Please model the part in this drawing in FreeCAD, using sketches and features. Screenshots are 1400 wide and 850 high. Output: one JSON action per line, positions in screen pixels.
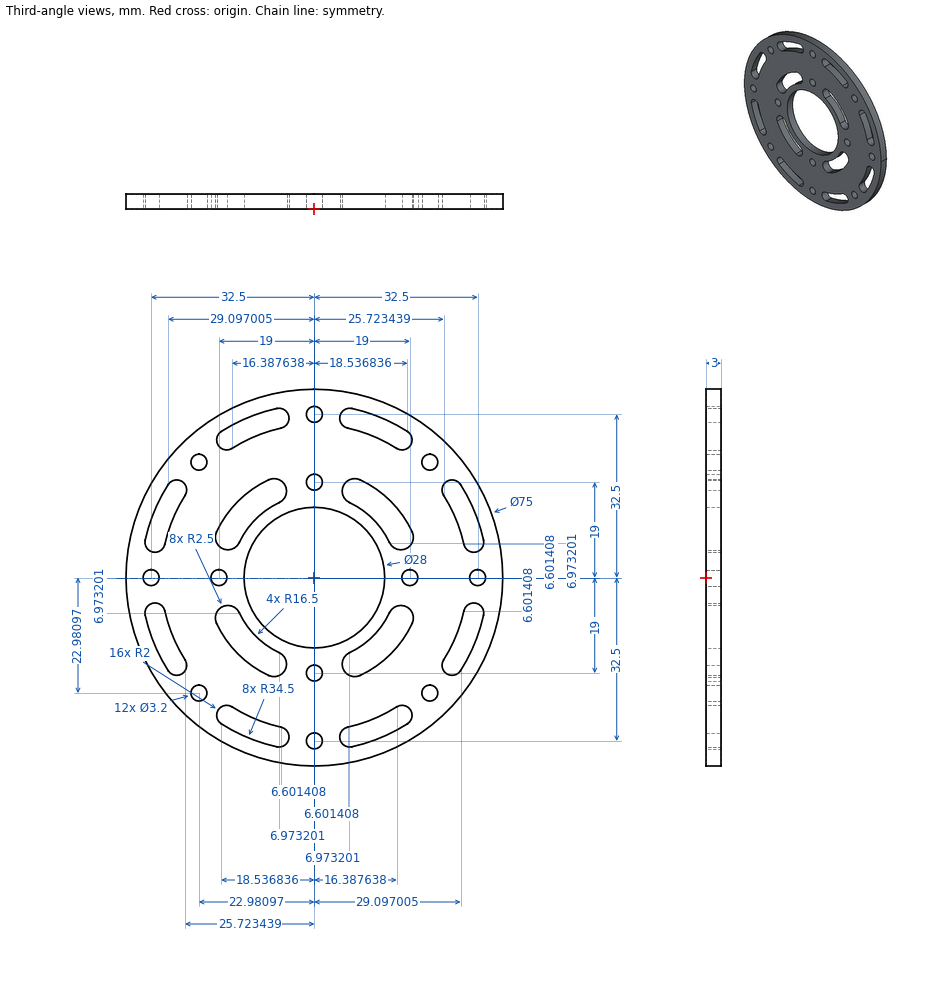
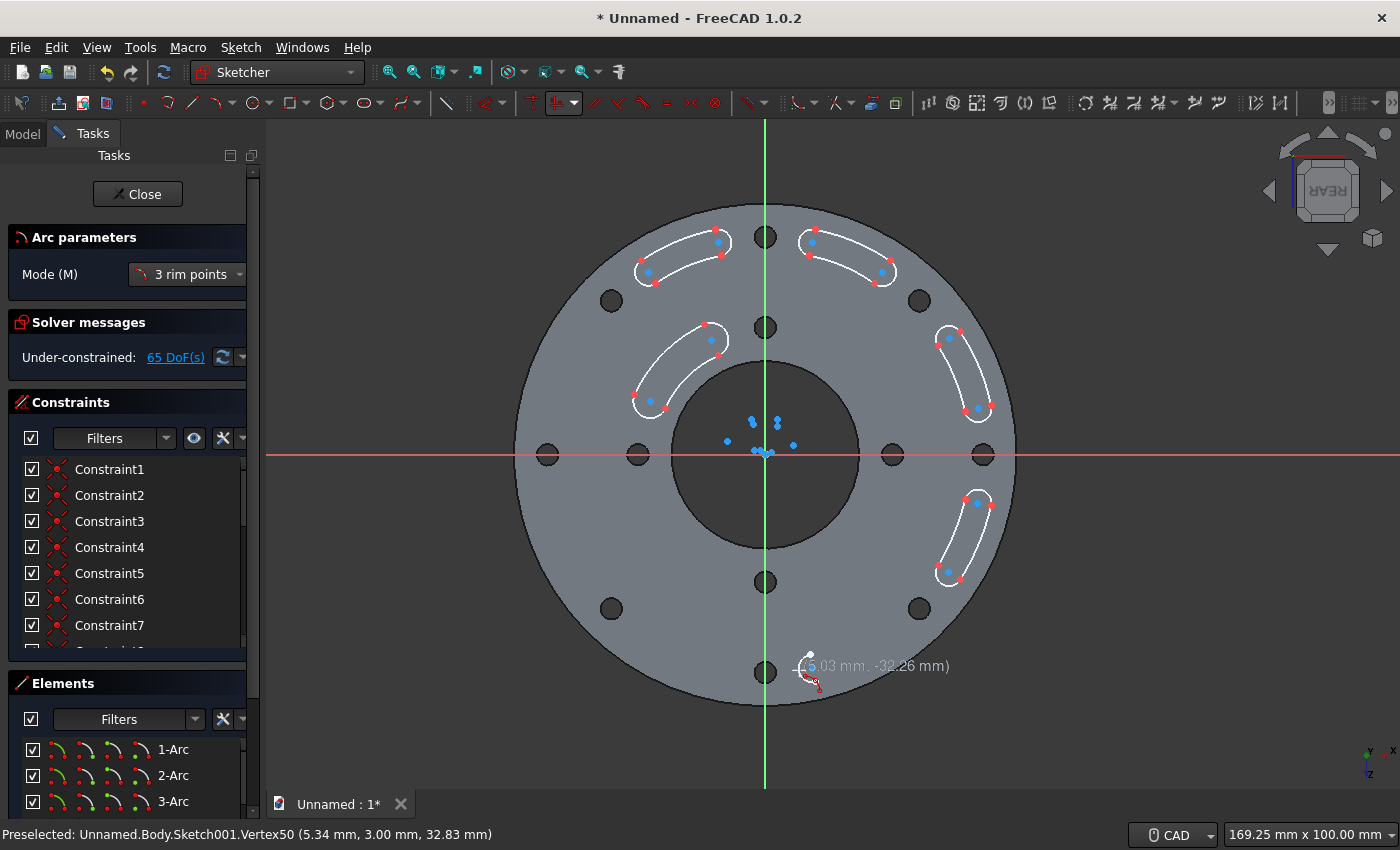
{"action": "left_click", "coordinate": [815, 682]}
{"action": "left_click", "coordinate": [890, 650]}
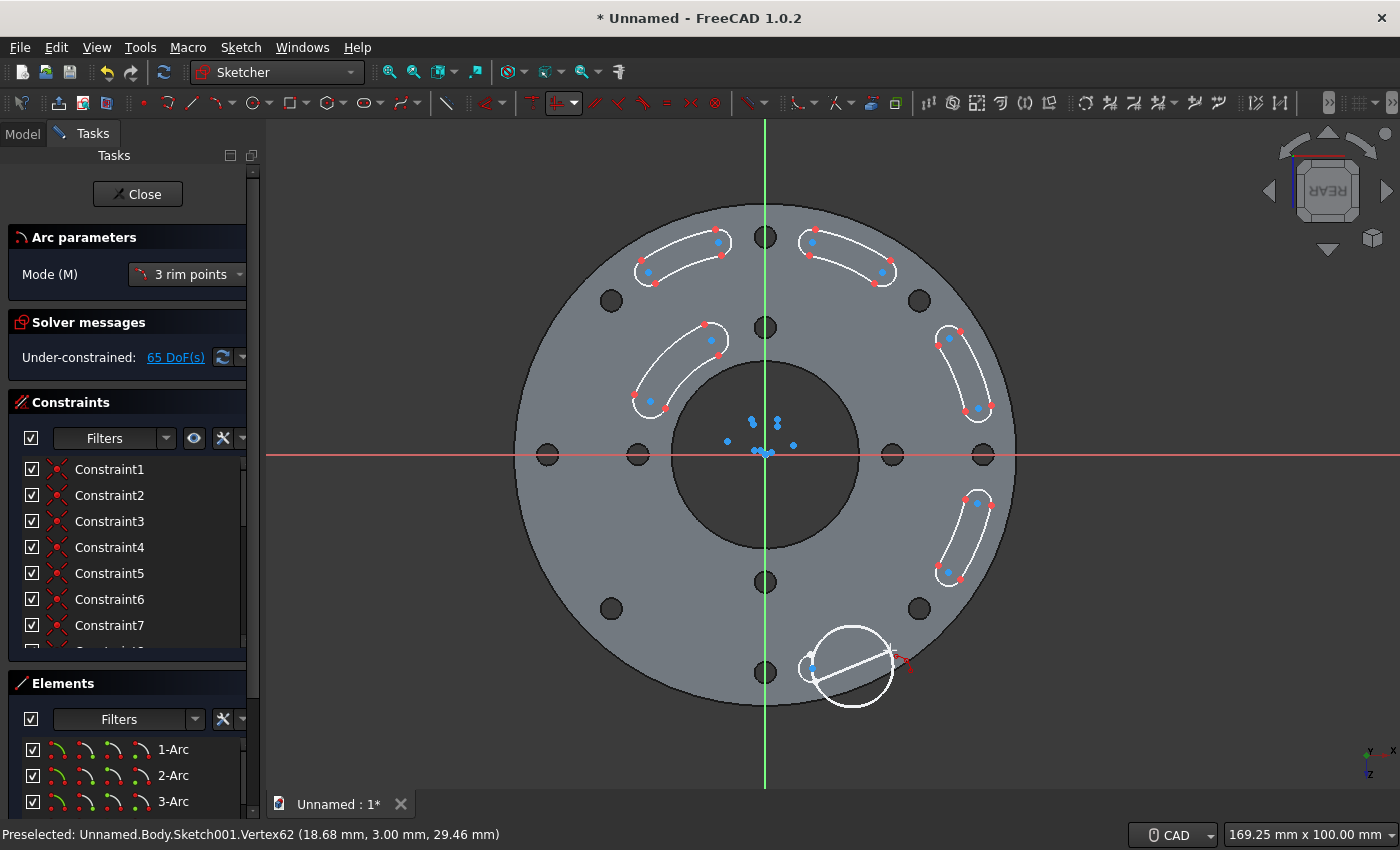
{"action": "scroll", "coordinate": [854, 668], "scroll_direction": "up", "scroll_amount": 8}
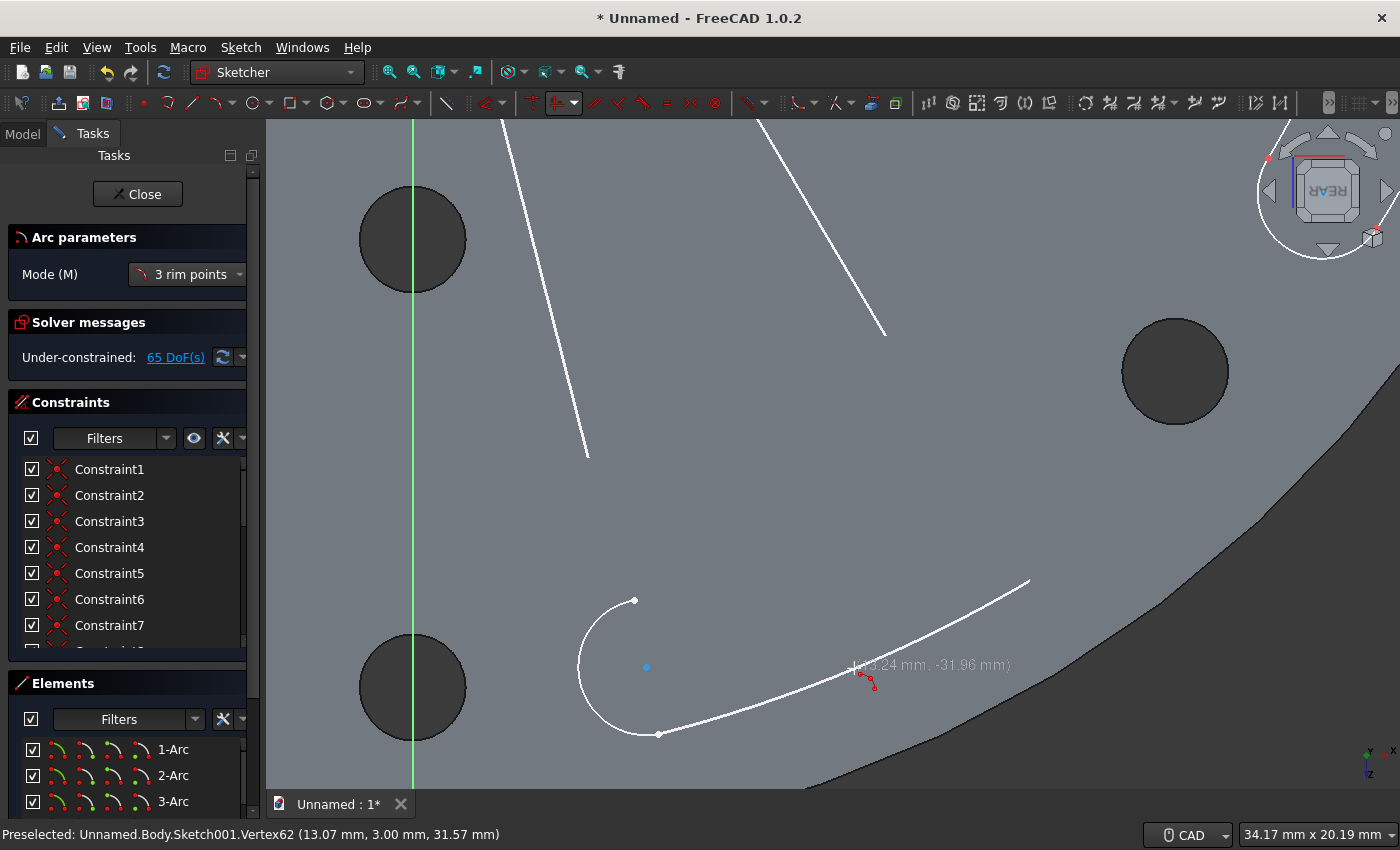
{"action": "left_click", "coordinate": [851, 667]}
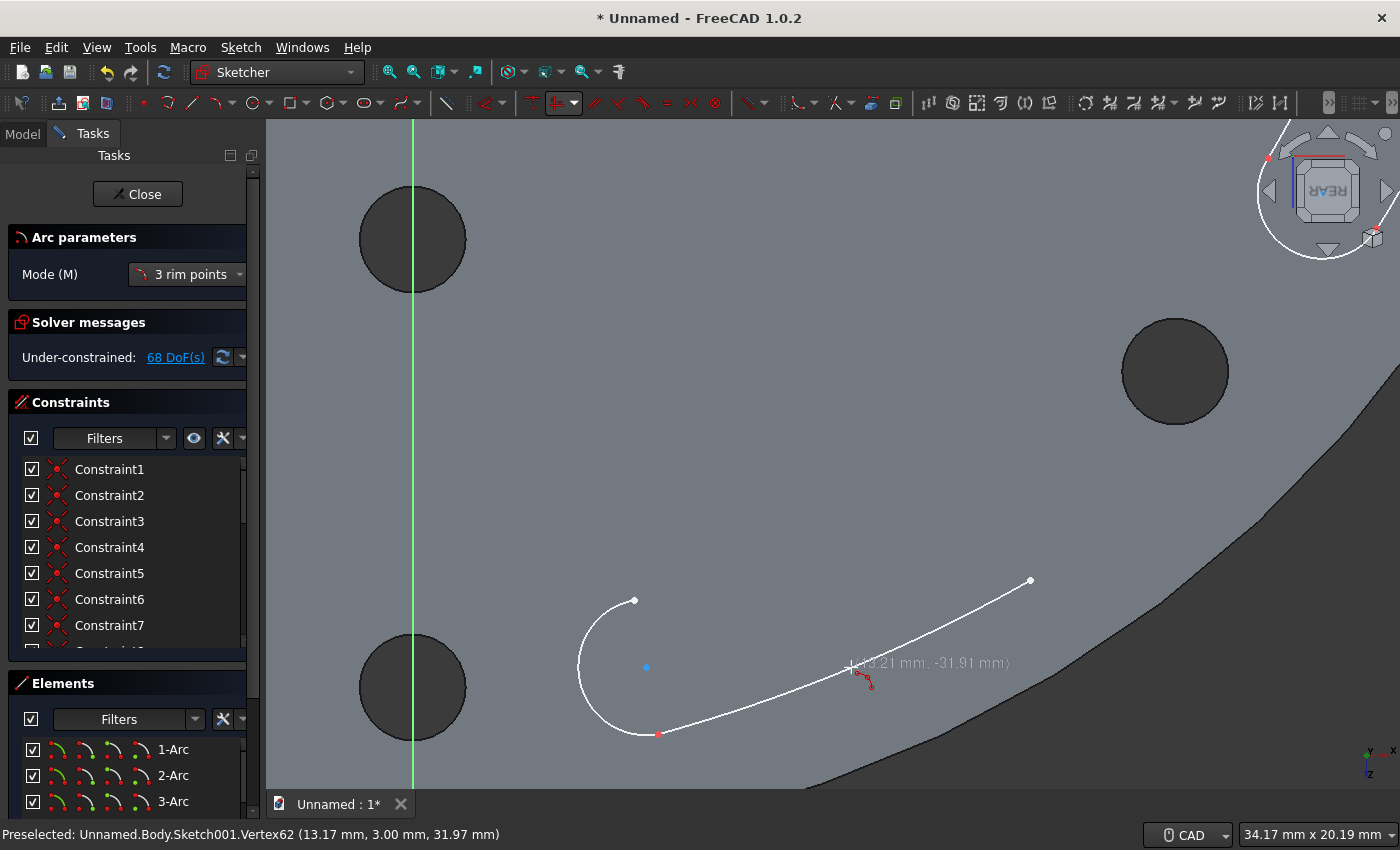
{"action": "scroll", "coordinate": [854, 668], "scroll_direction": "down", "scroll_amount": 8}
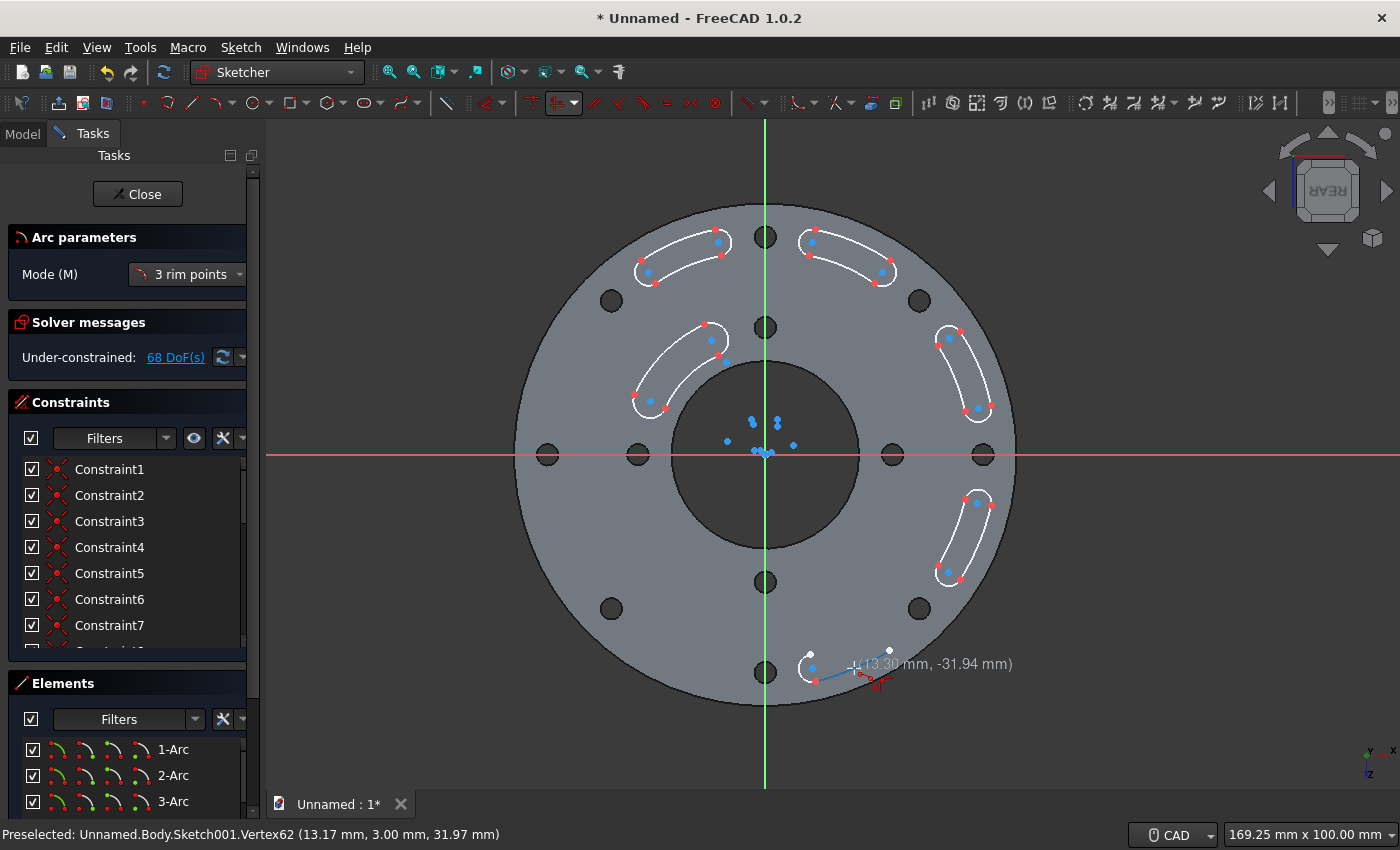
{"action": "left_click", "coordinate": [890, 651]}
{"action": "left_click", "coordinate": [875, 627]}
{"action": "left_click", "coordinate": [894, 631]}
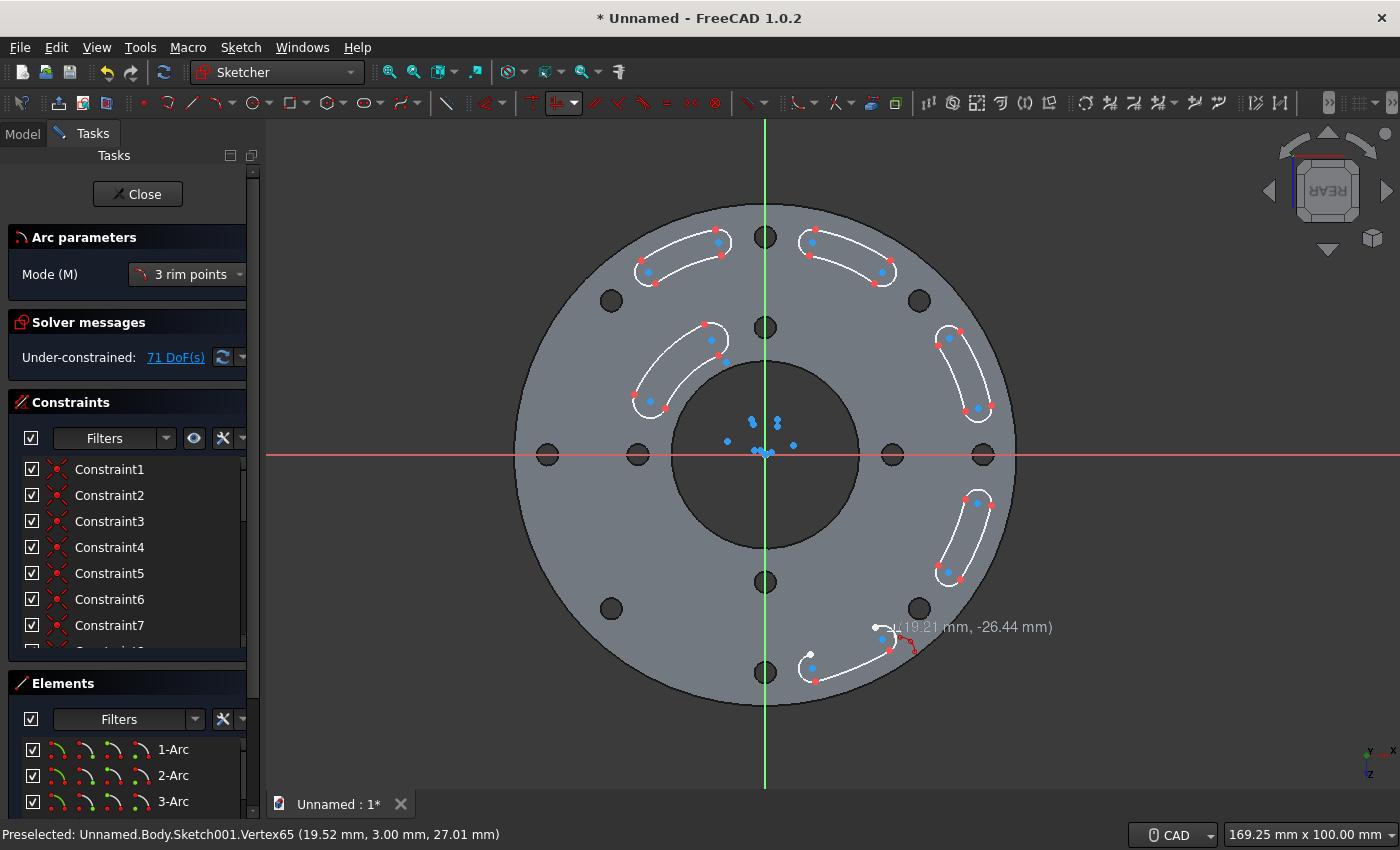
{"action": "left_click", "coordinate": [875, 628]}
{"action": "left_click", "coordinate": [810, 655]}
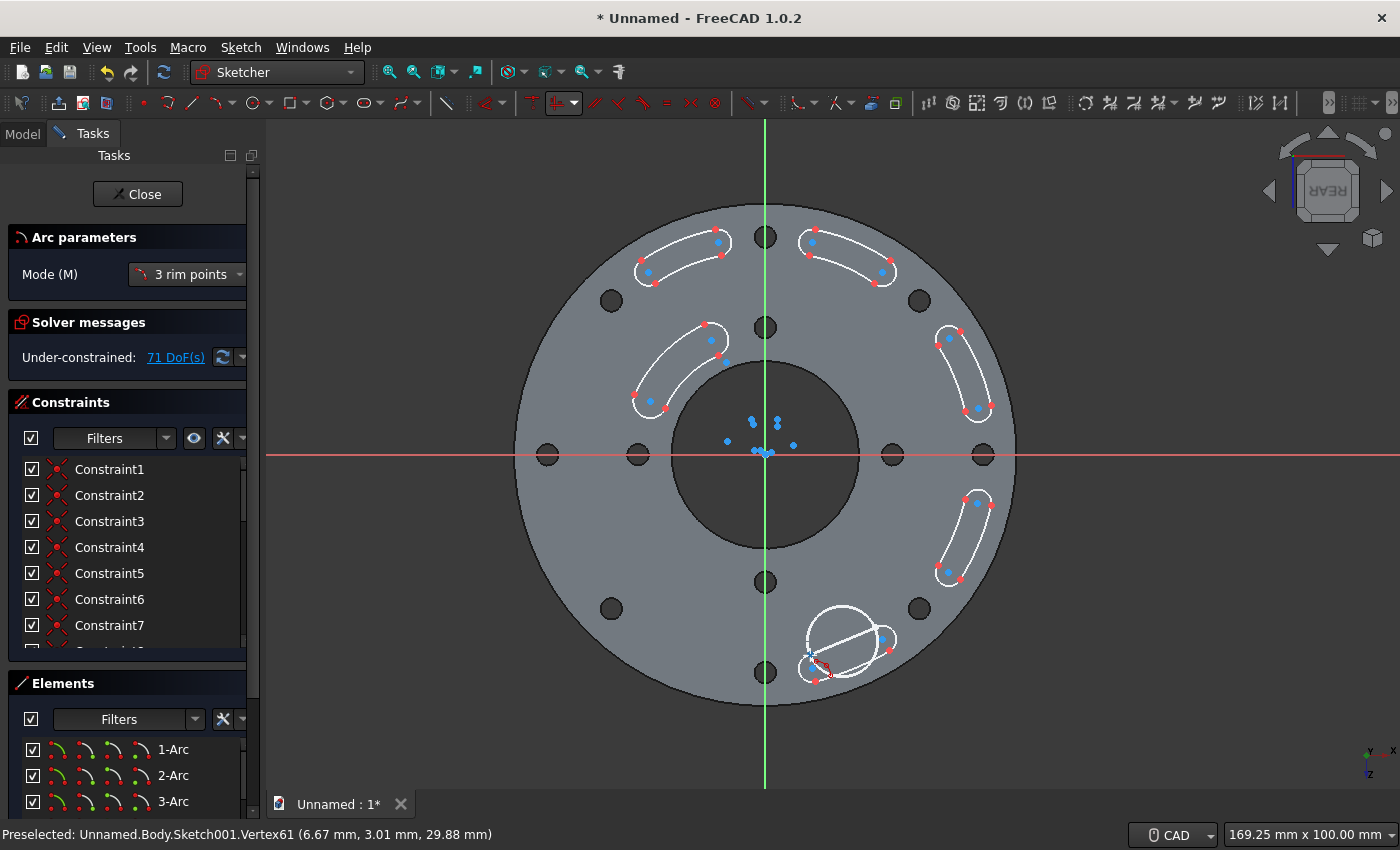
{"action": "scroll", "coordinate": [844, 644], "scroll_direction": "up", "scroll_amount": 9}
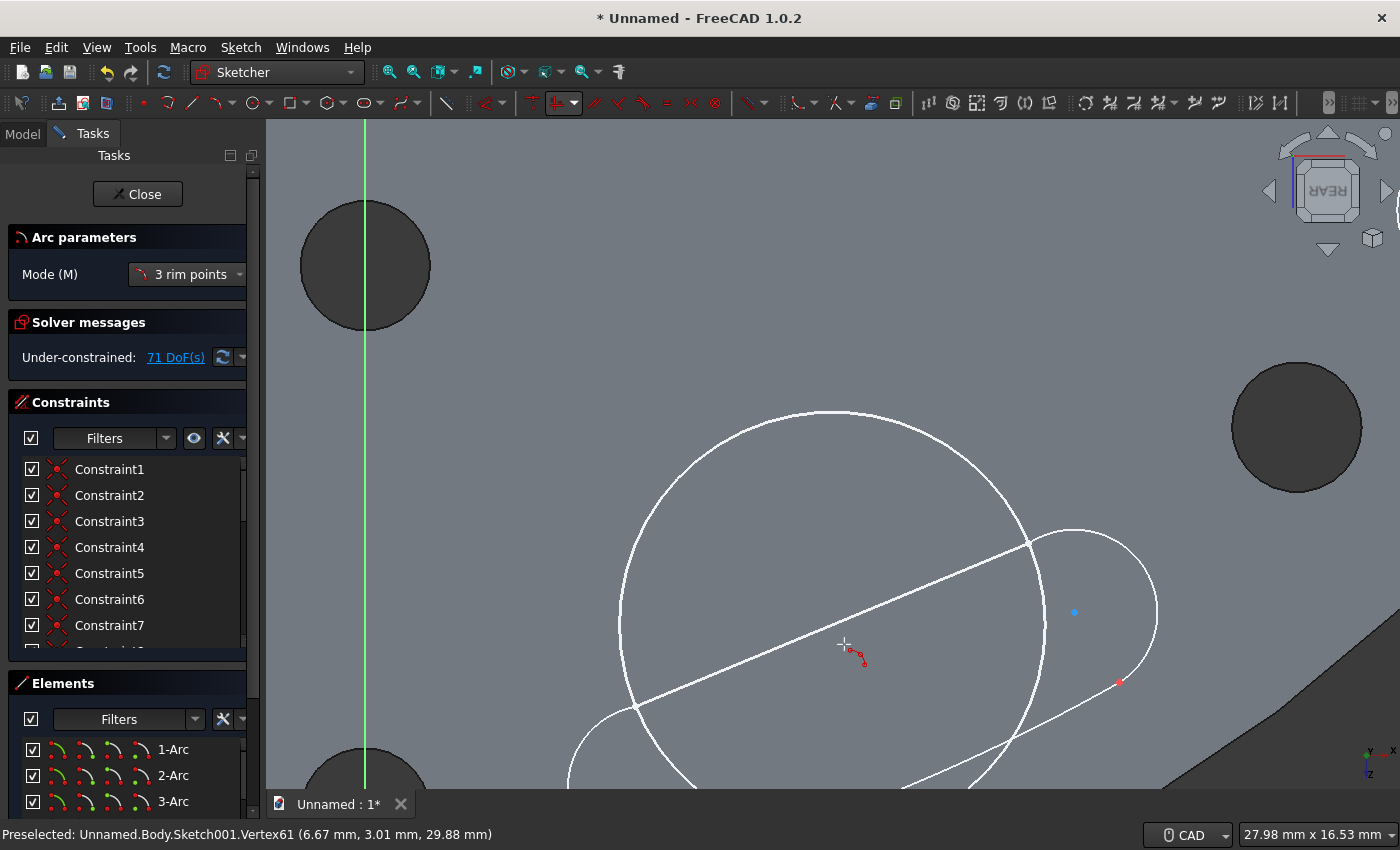
{"action": "left_click", "coordinate": [838, 638]}